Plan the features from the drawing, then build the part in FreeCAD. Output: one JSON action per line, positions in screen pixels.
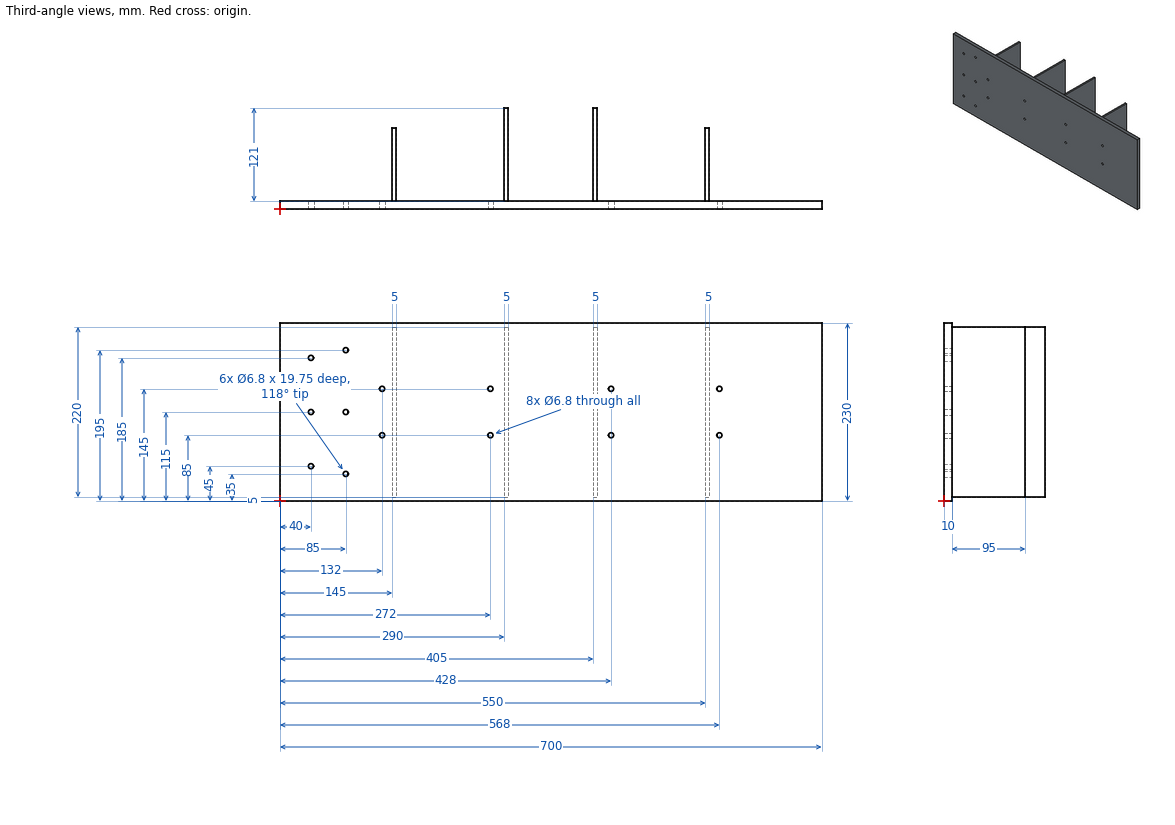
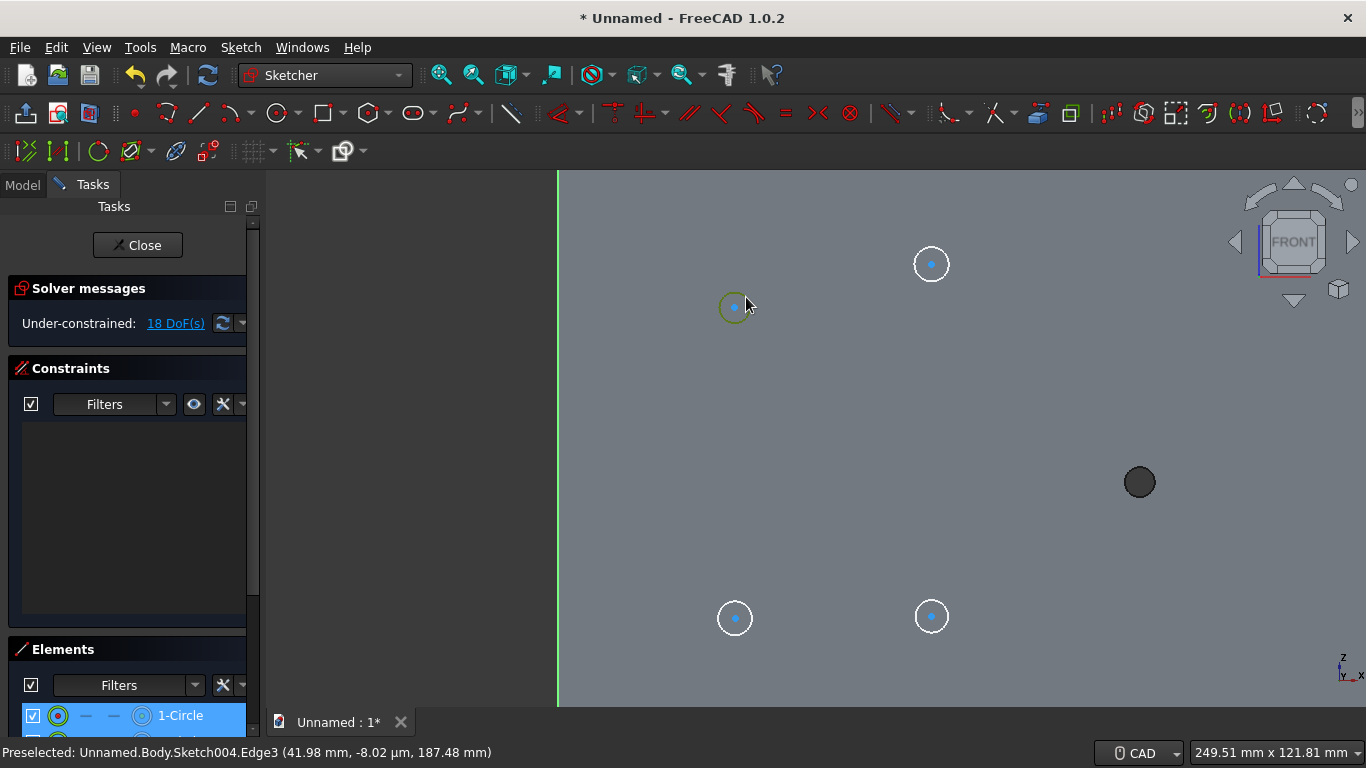
{"action": "left_click", "coordinate": [944, 252]}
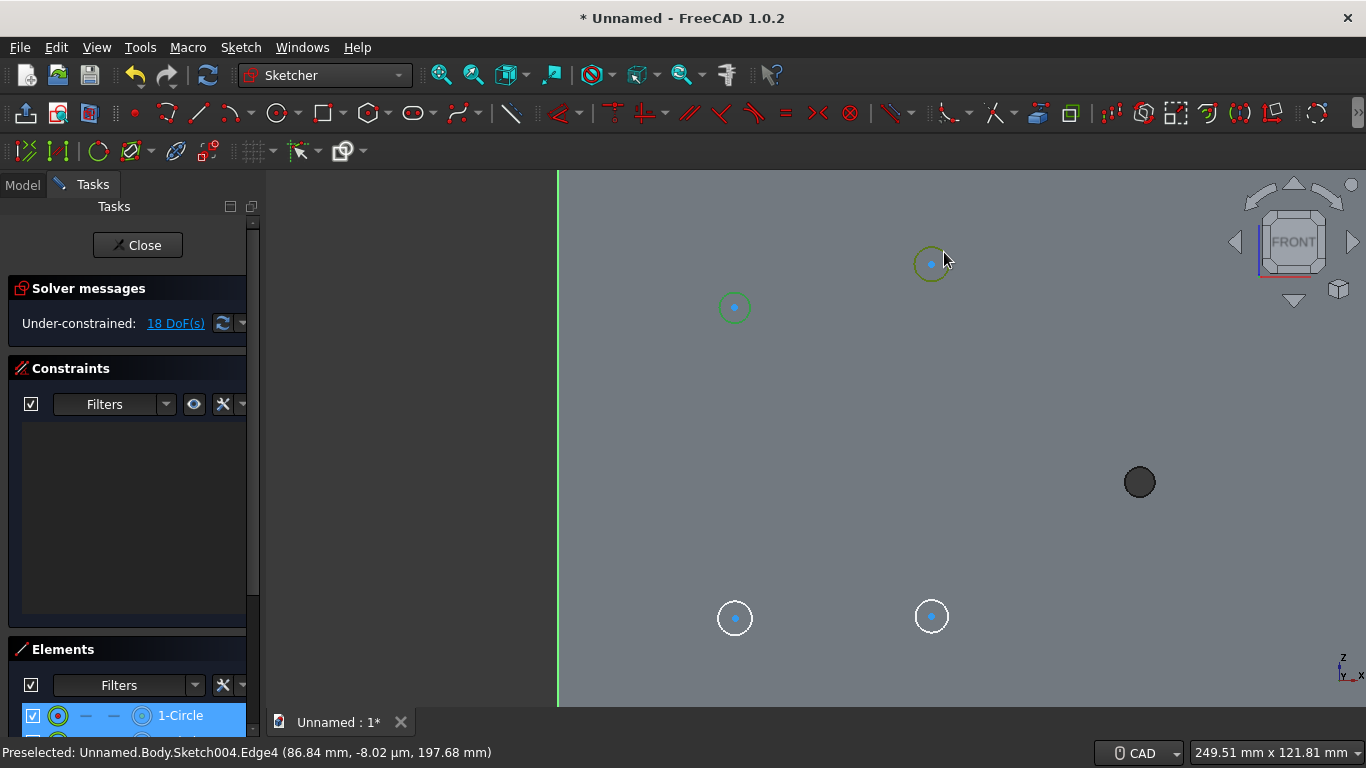
{"action": "left_click", "coordinate": [747, 606]}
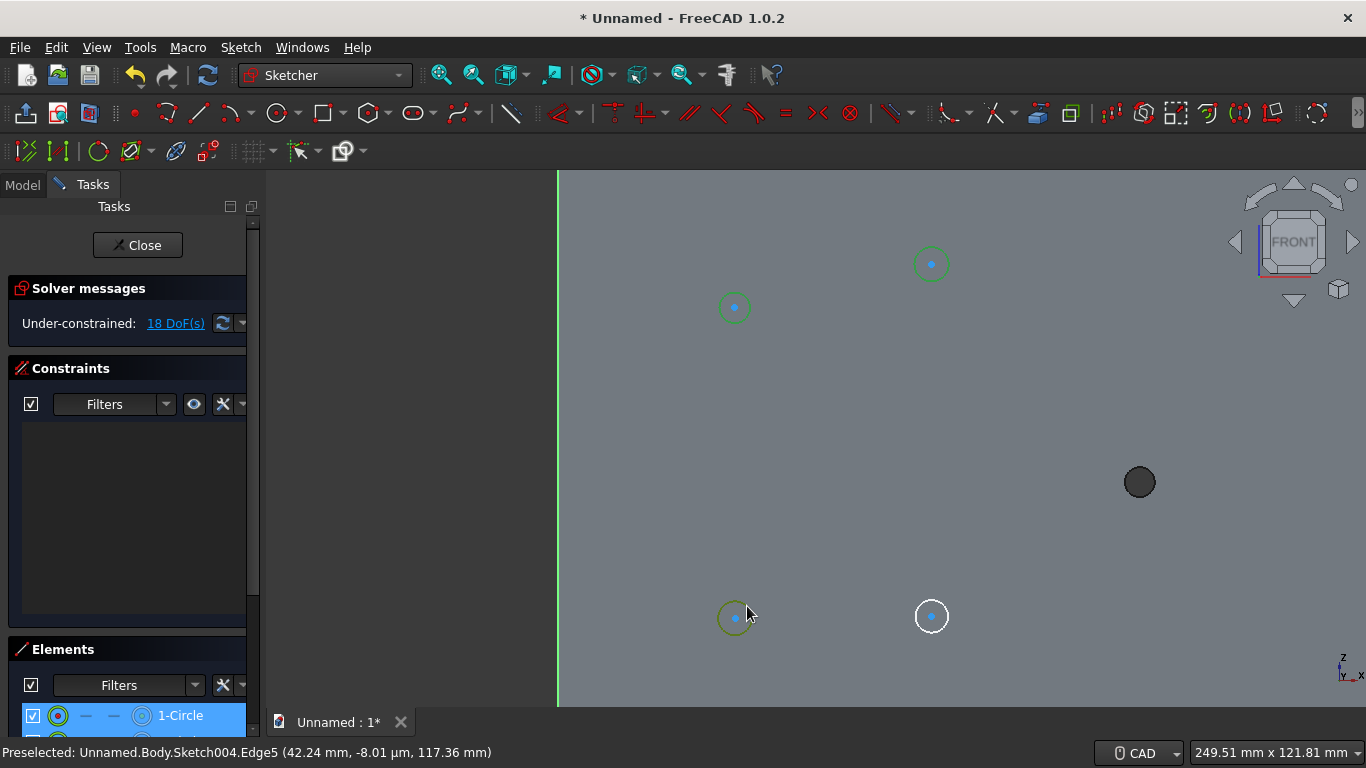
{"action": "left_click", "coordinate": [943, 605]}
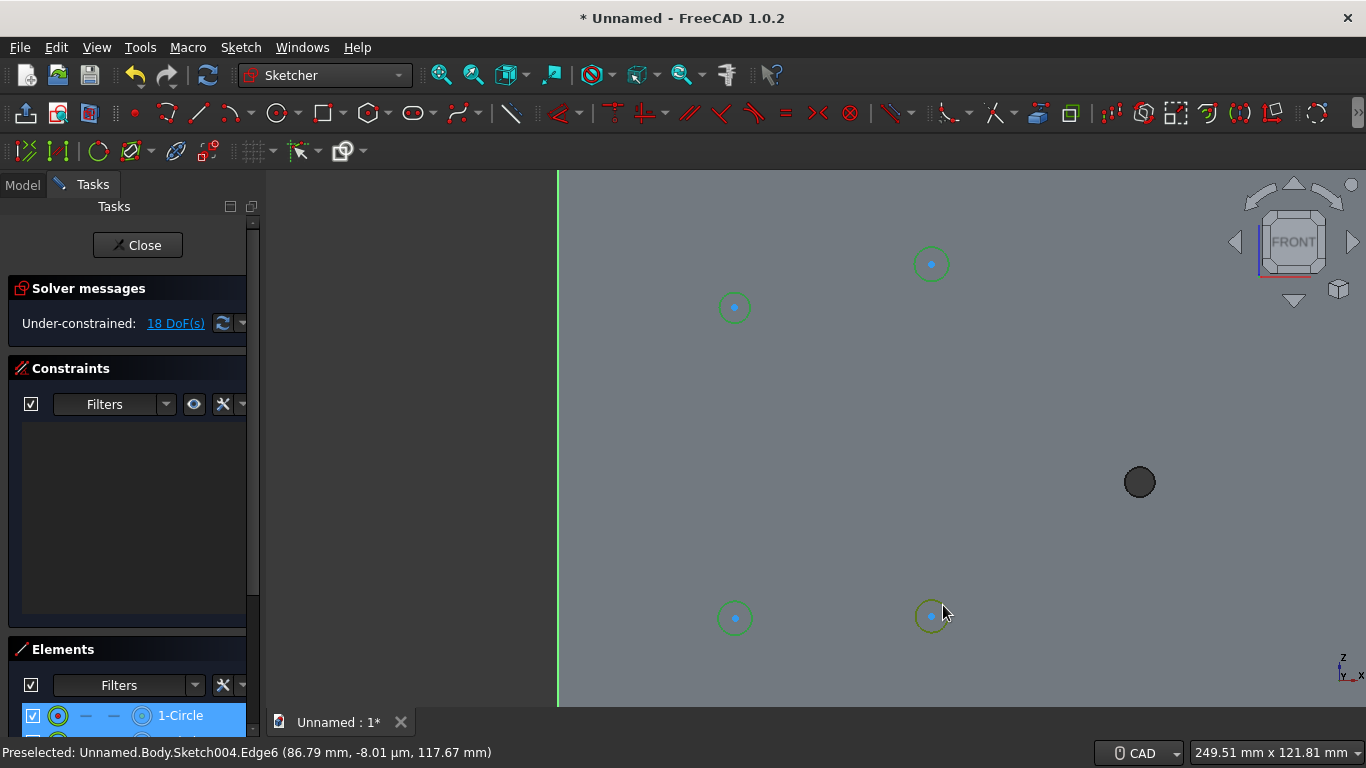
{"action": "left_click", "coordinate": [786, 114]}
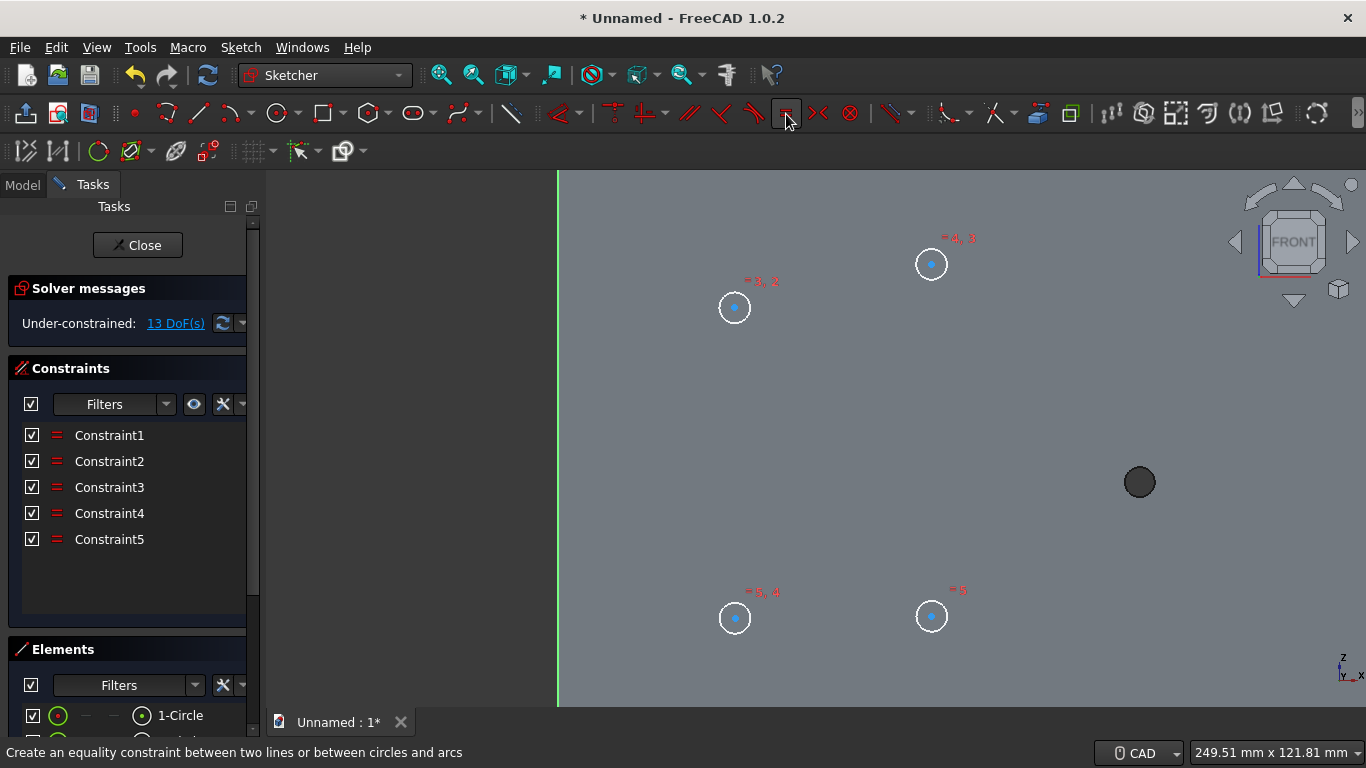
{"action": "left_click", "coordinate": [558, 114]}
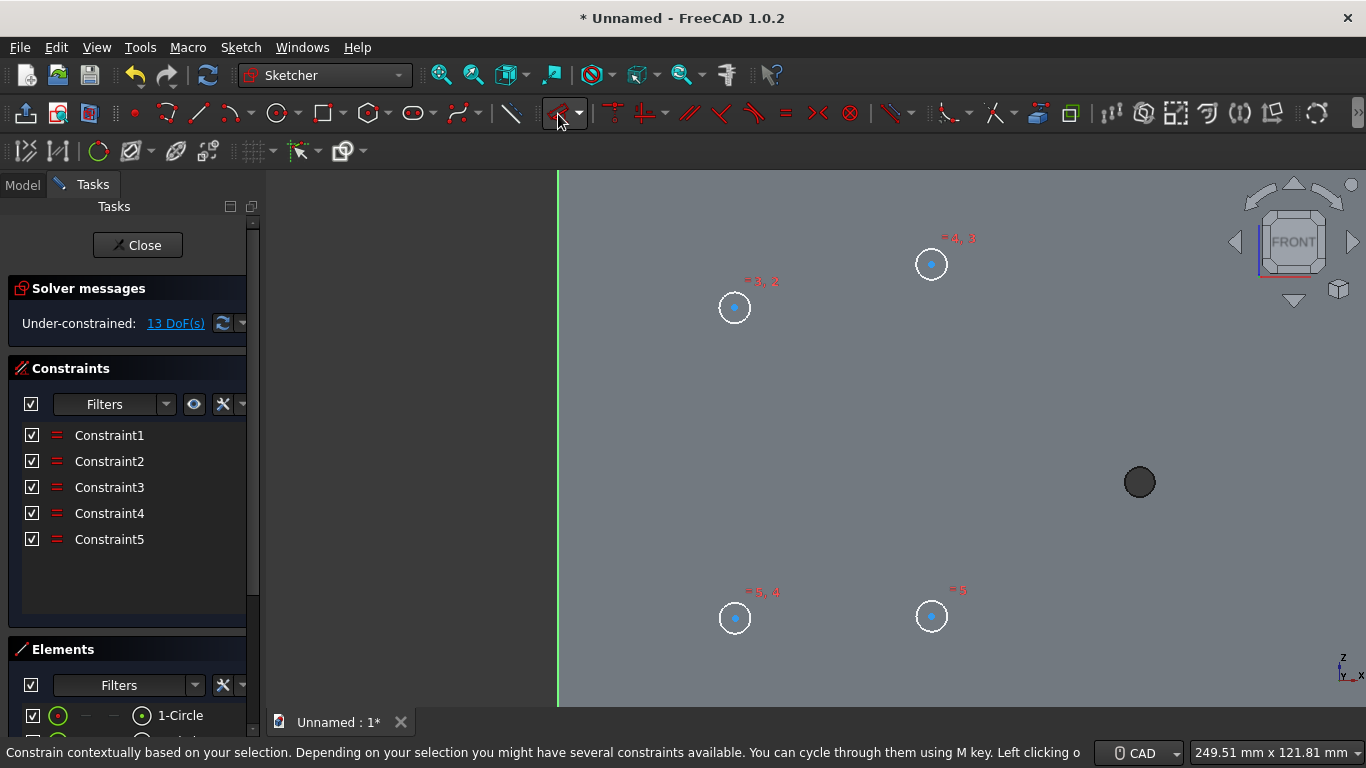
{"action": "scroll", "coordinate": [744, 296], "scroll_direction": "down", "scroll_amount": 5}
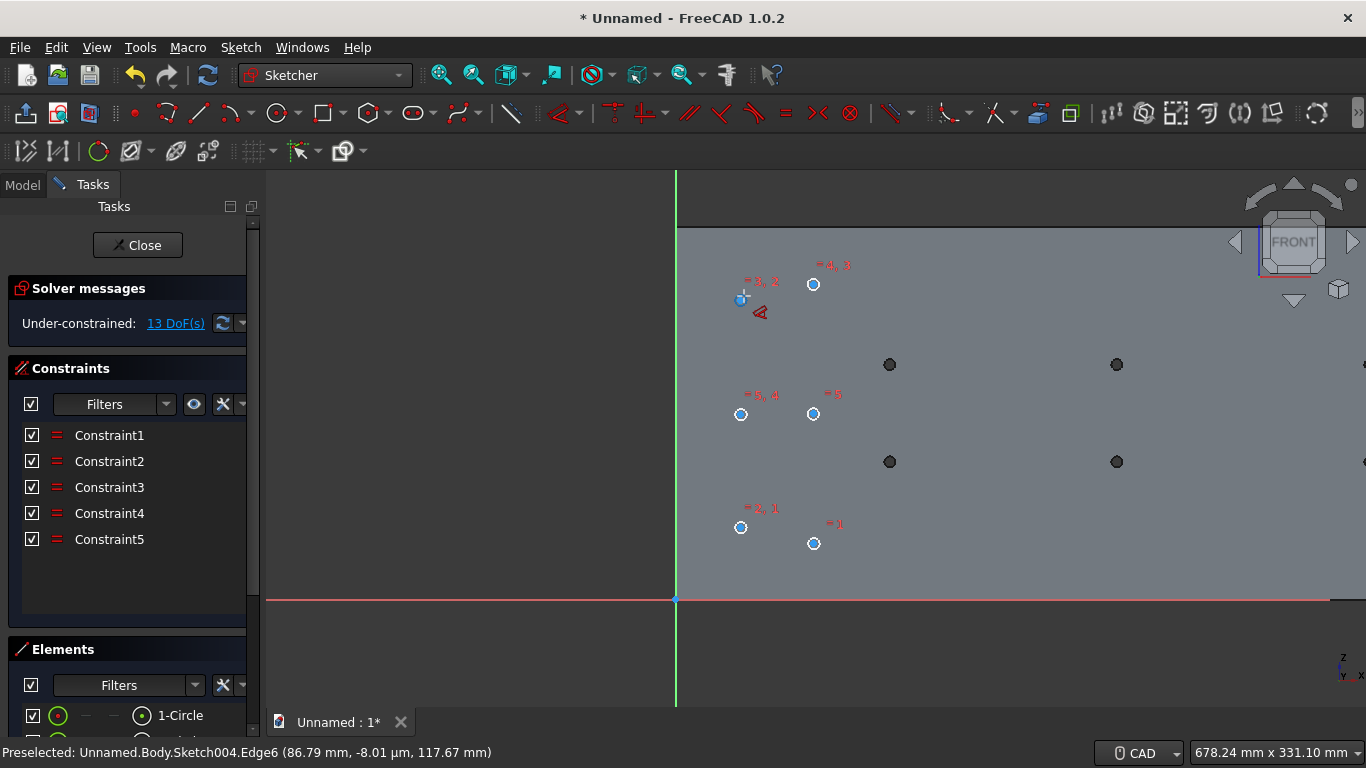
{"action": "scroll", "coordinate": [818, 540], "scroll_direction": "up", "scroll_amount": 7}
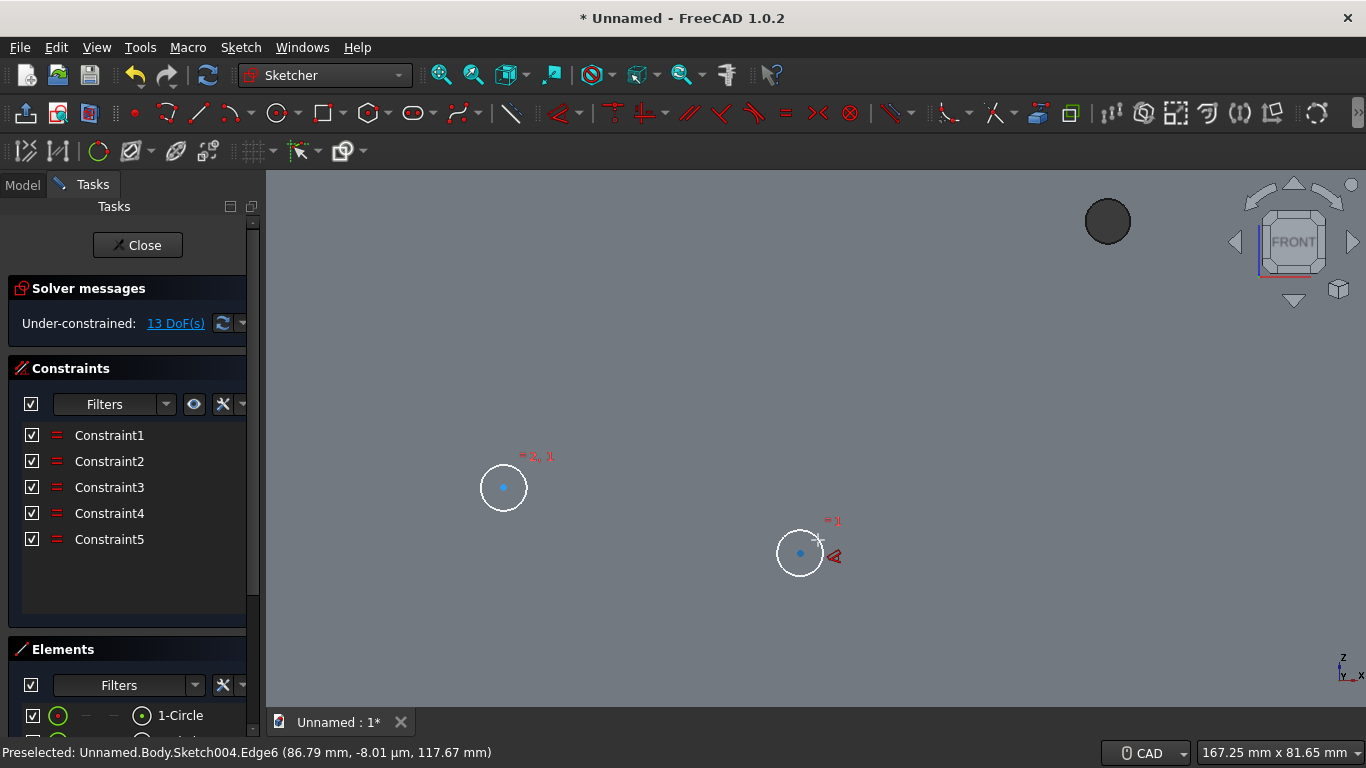
{"action": "left_click", "coordinate": [816, 537]}
{"action": "left_click", "coordinate": [838, 514]}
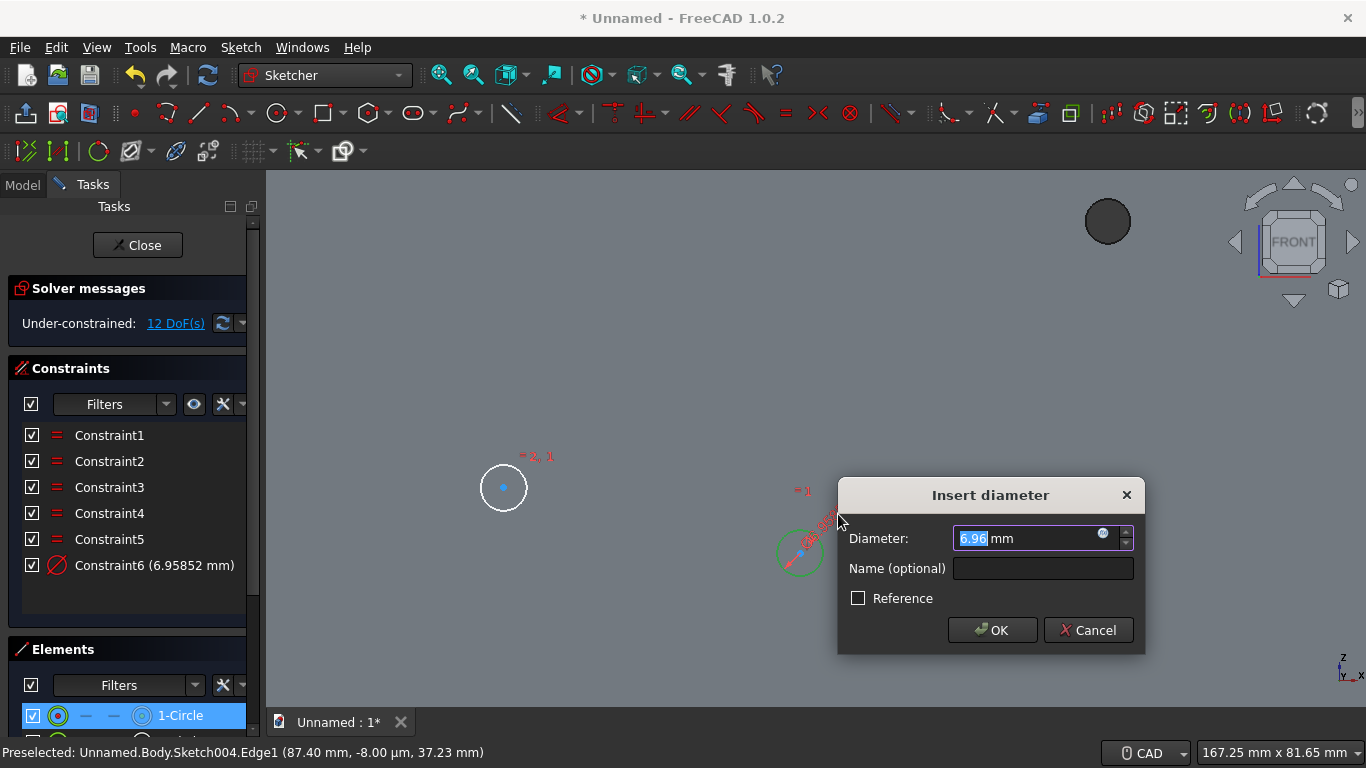
{"action": "type", "text": "6.8"}
{"action": "key", "text": "Return"}